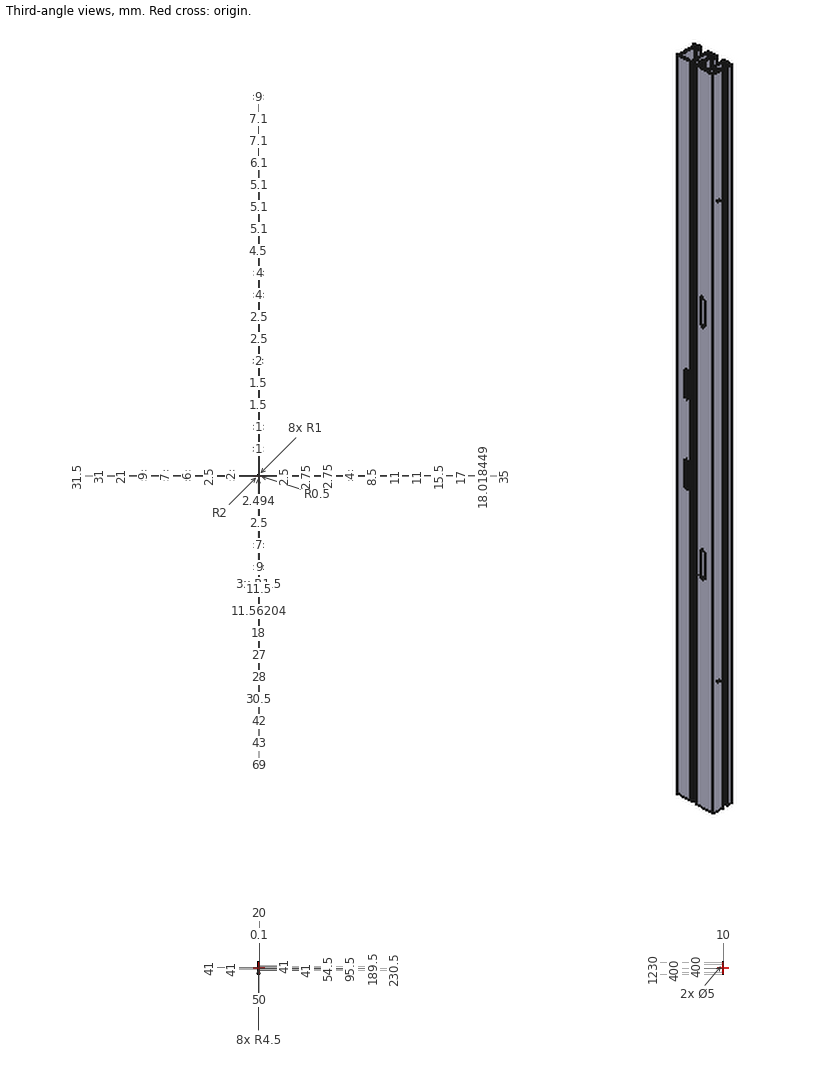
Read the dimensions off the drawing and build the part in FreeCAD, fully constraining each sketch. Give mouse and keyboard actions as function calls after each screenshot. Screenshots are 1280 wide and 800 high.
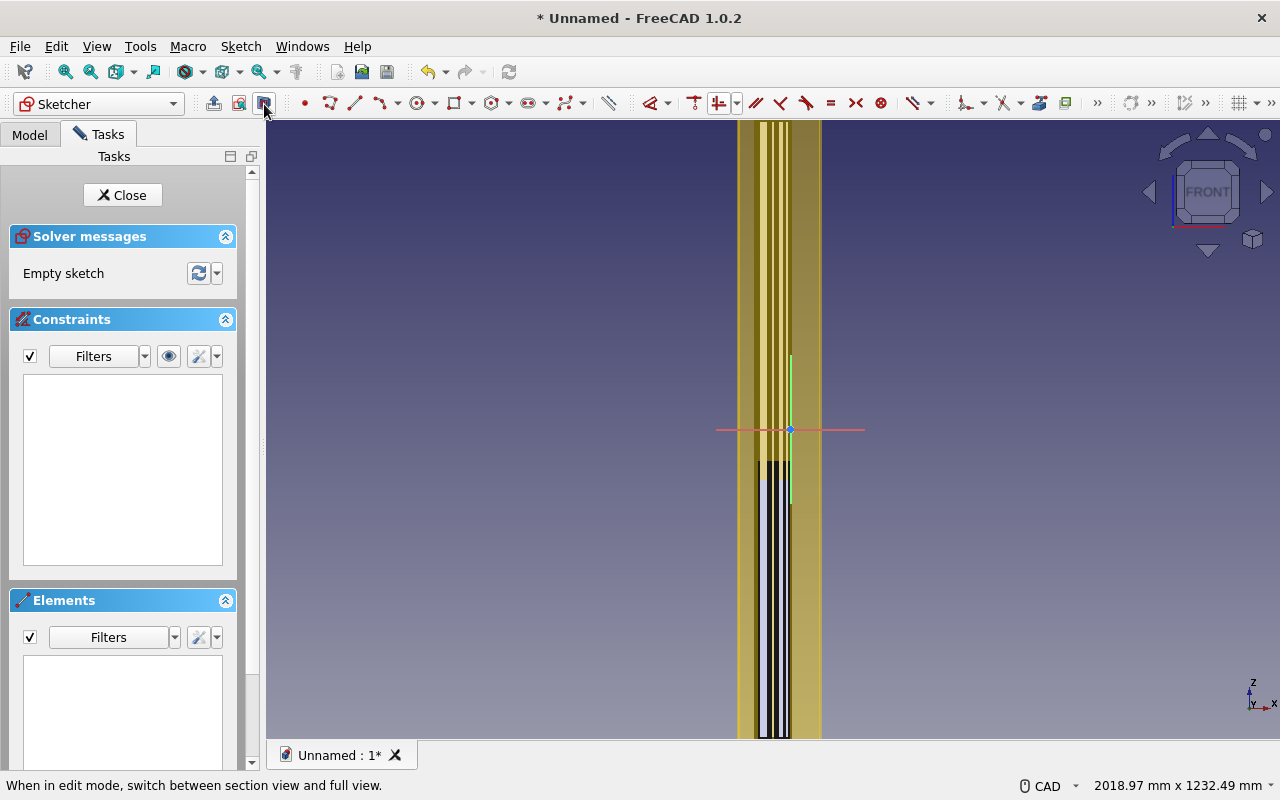
scroll(865, 430, up, 3)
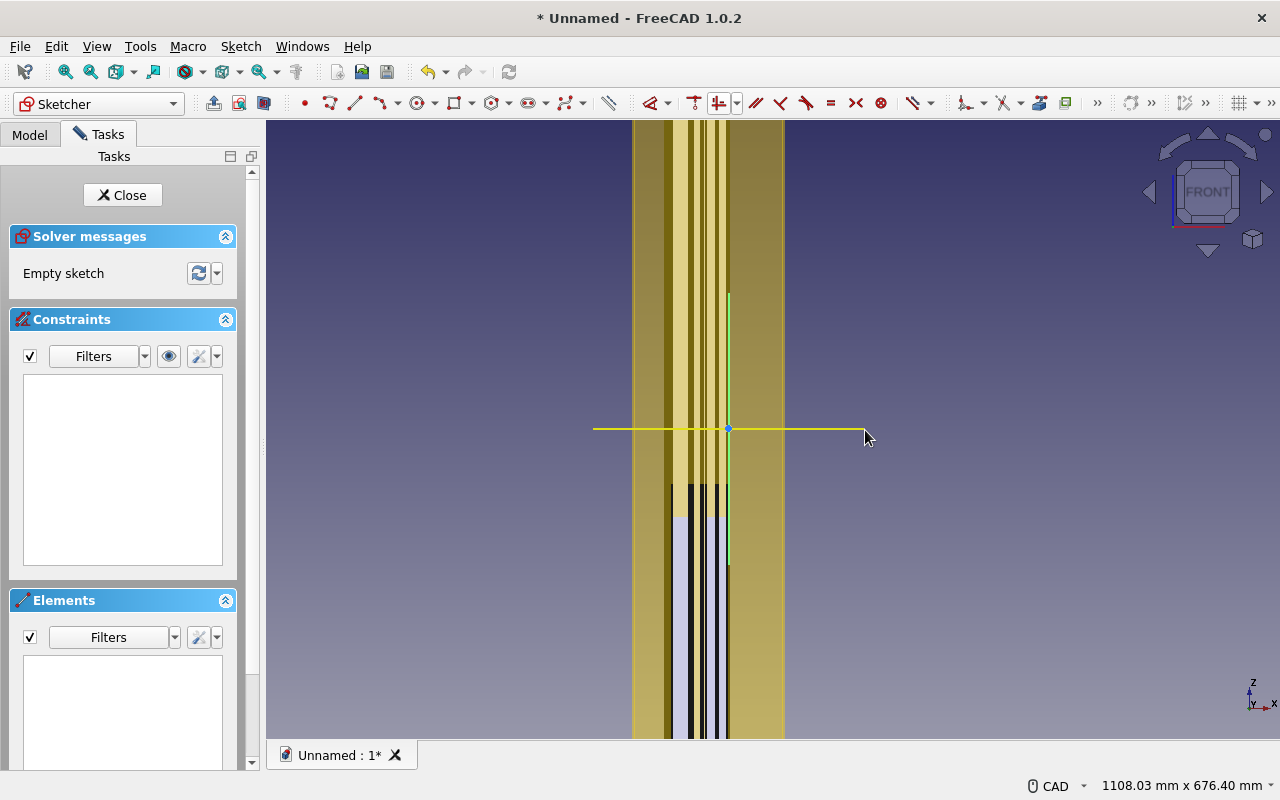
click(528, 104)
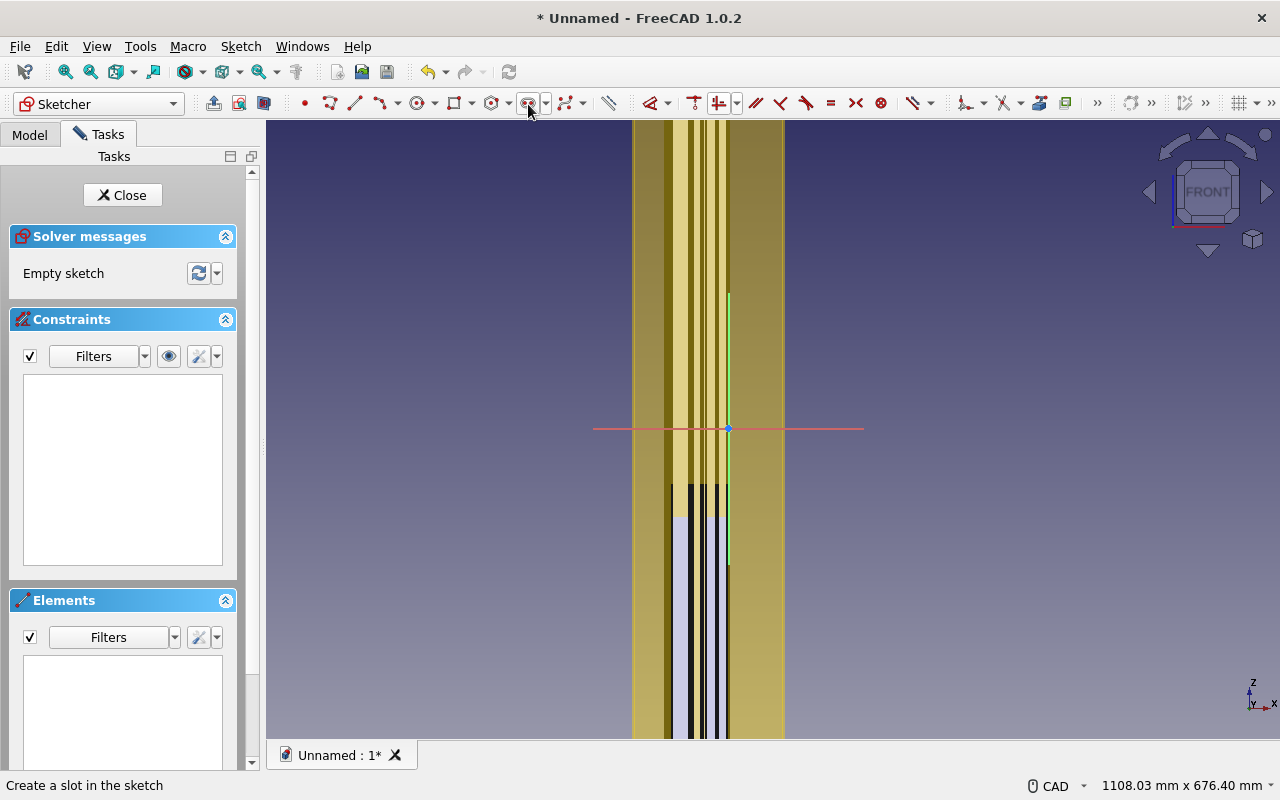
scroll(711, 255, up, 9)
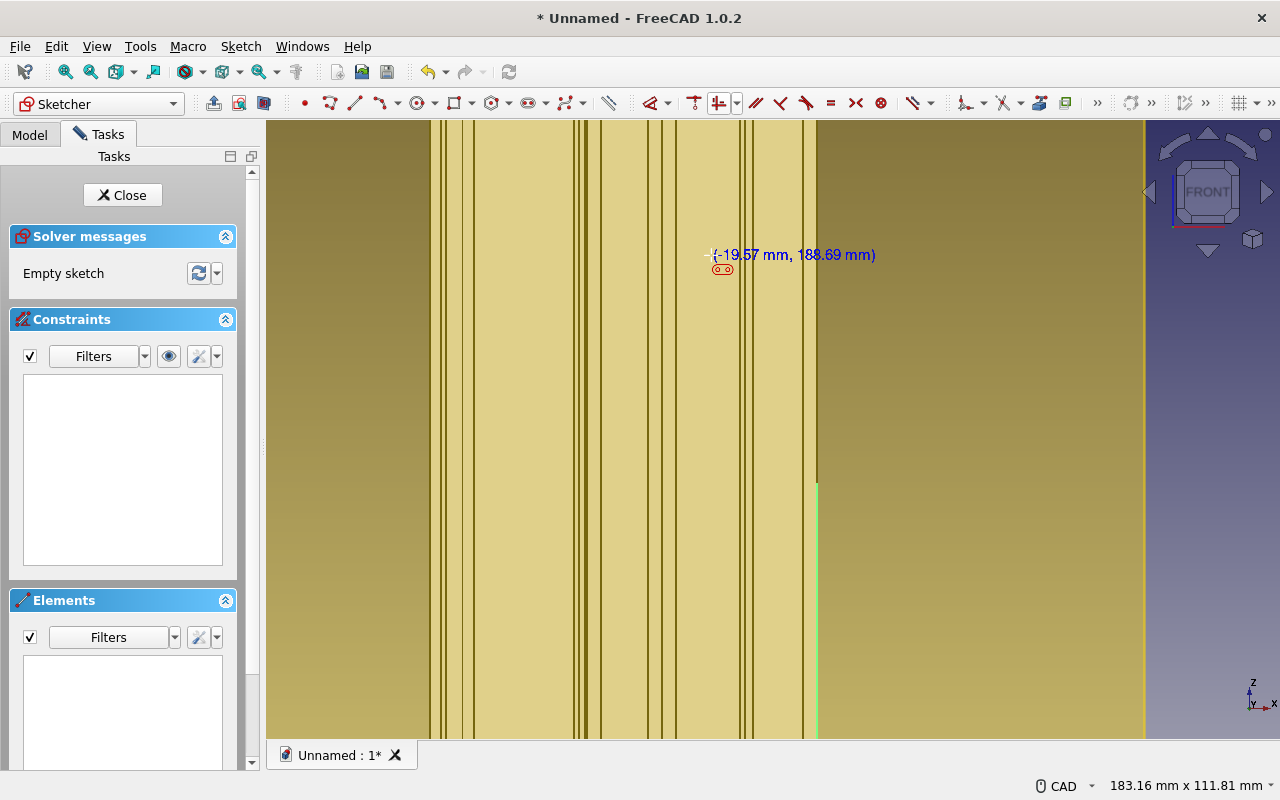
scroll(712, 256, down, 9)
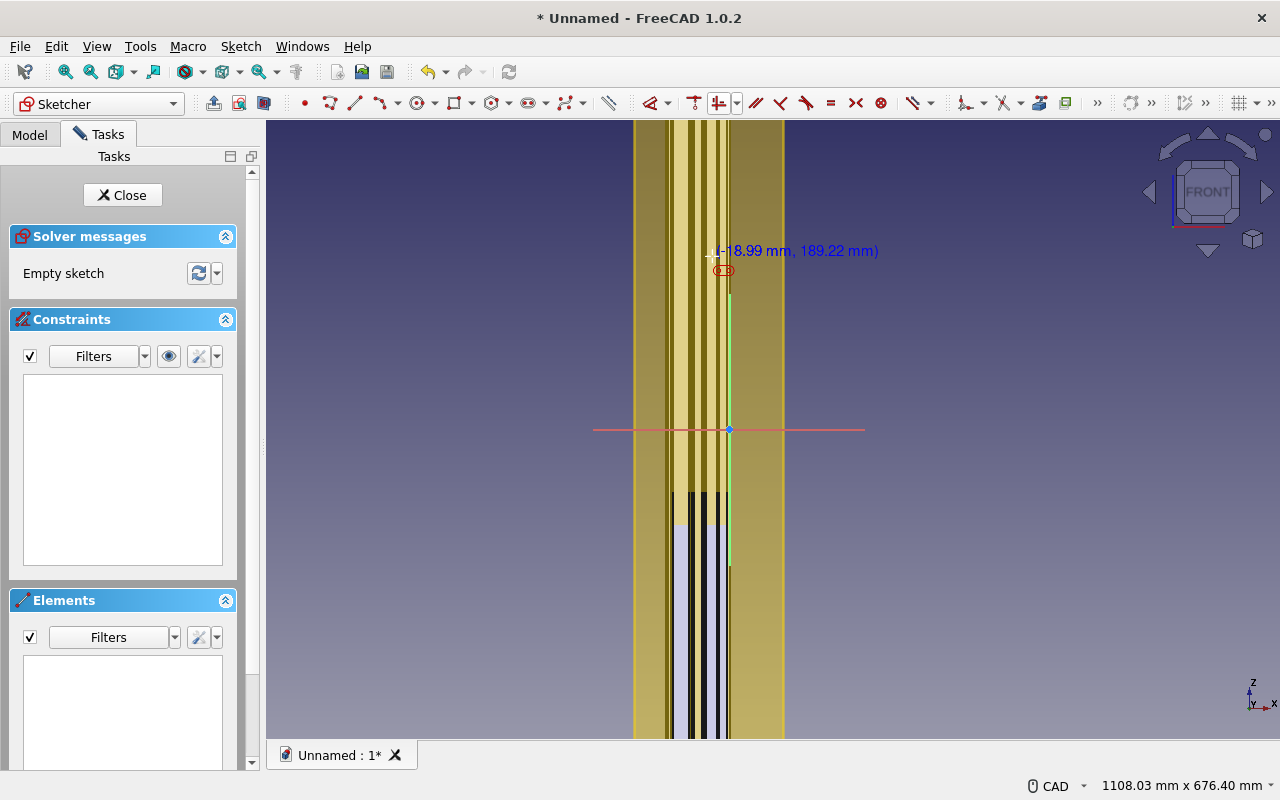
click(711, 256)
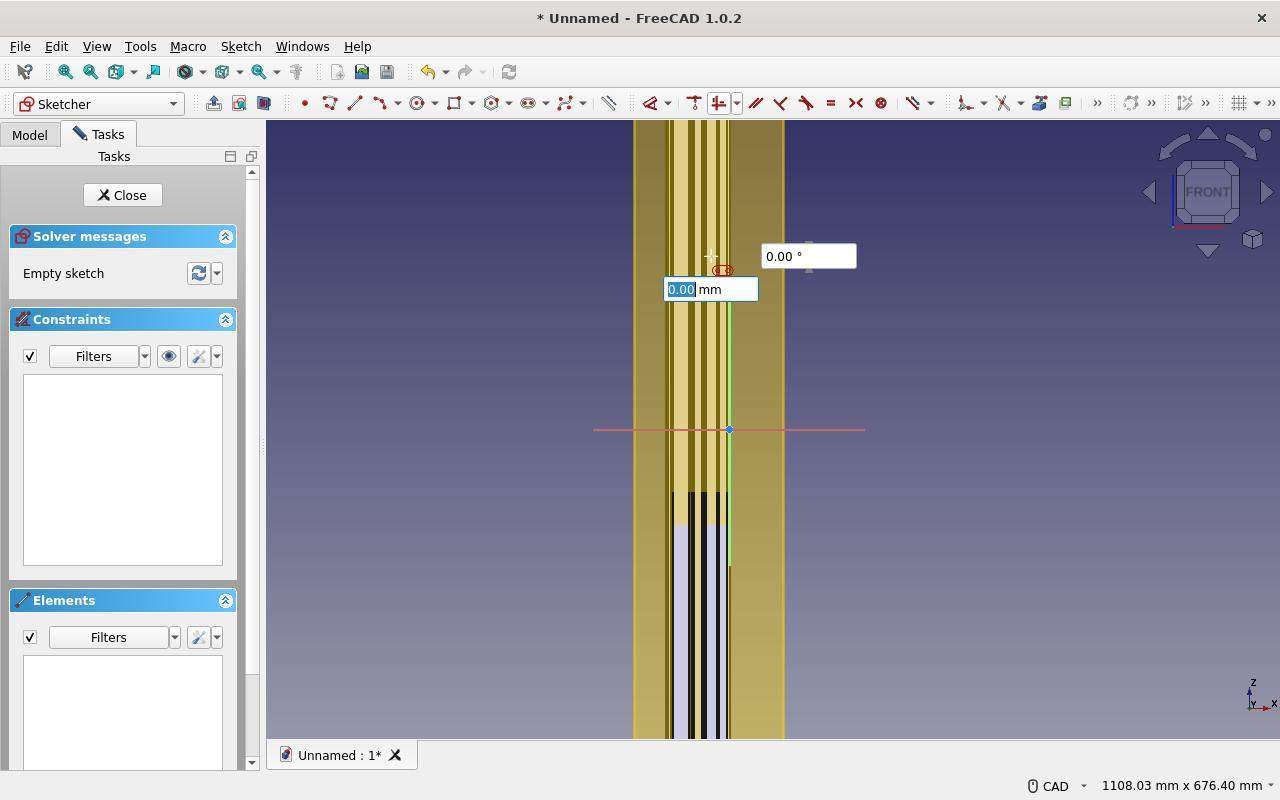
click(711, 219)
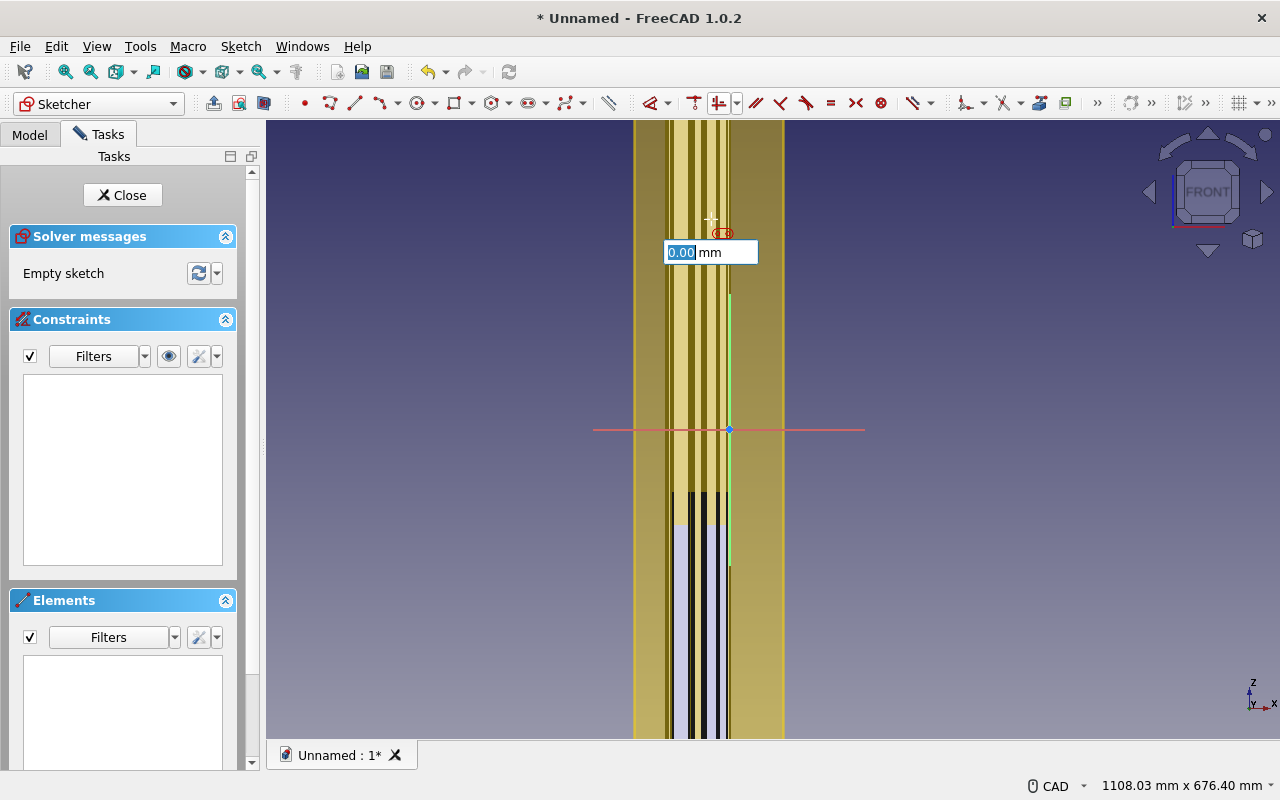
scroll(716, 237, up, 7)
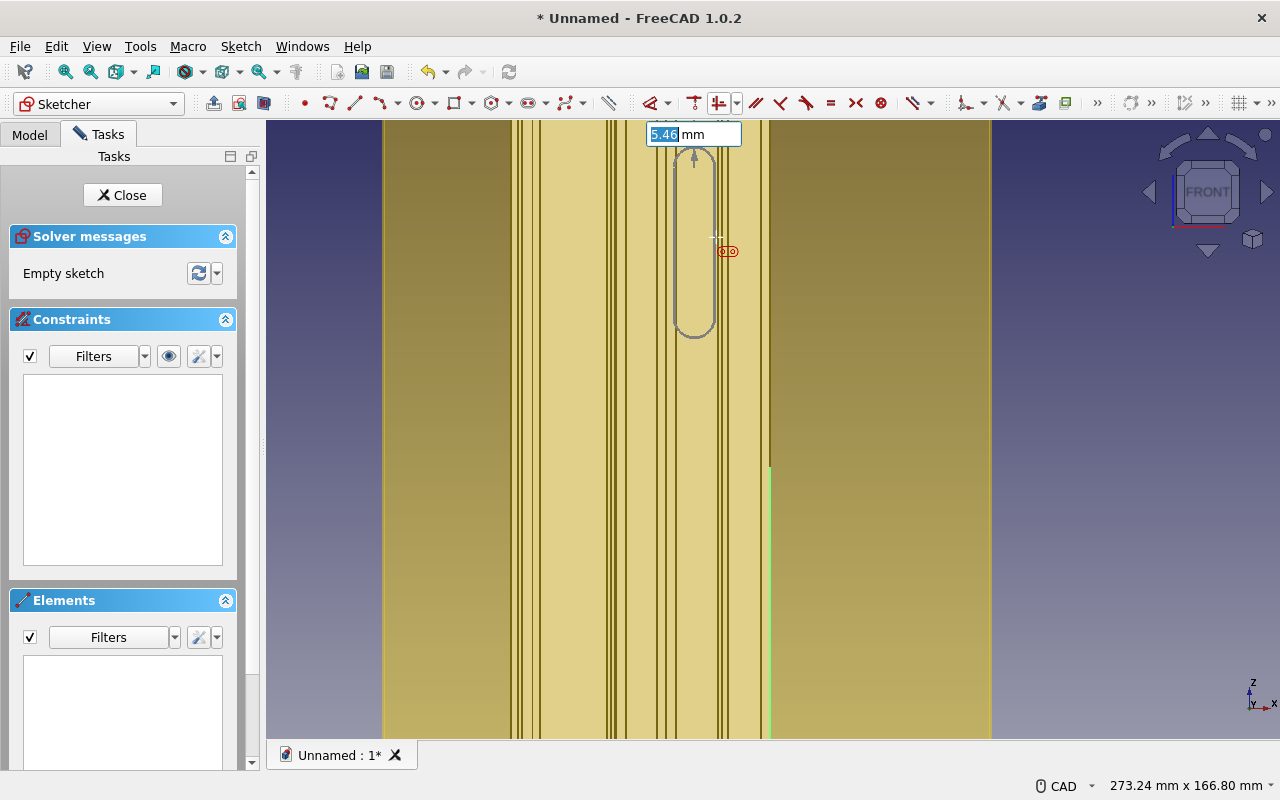
click(713, 238)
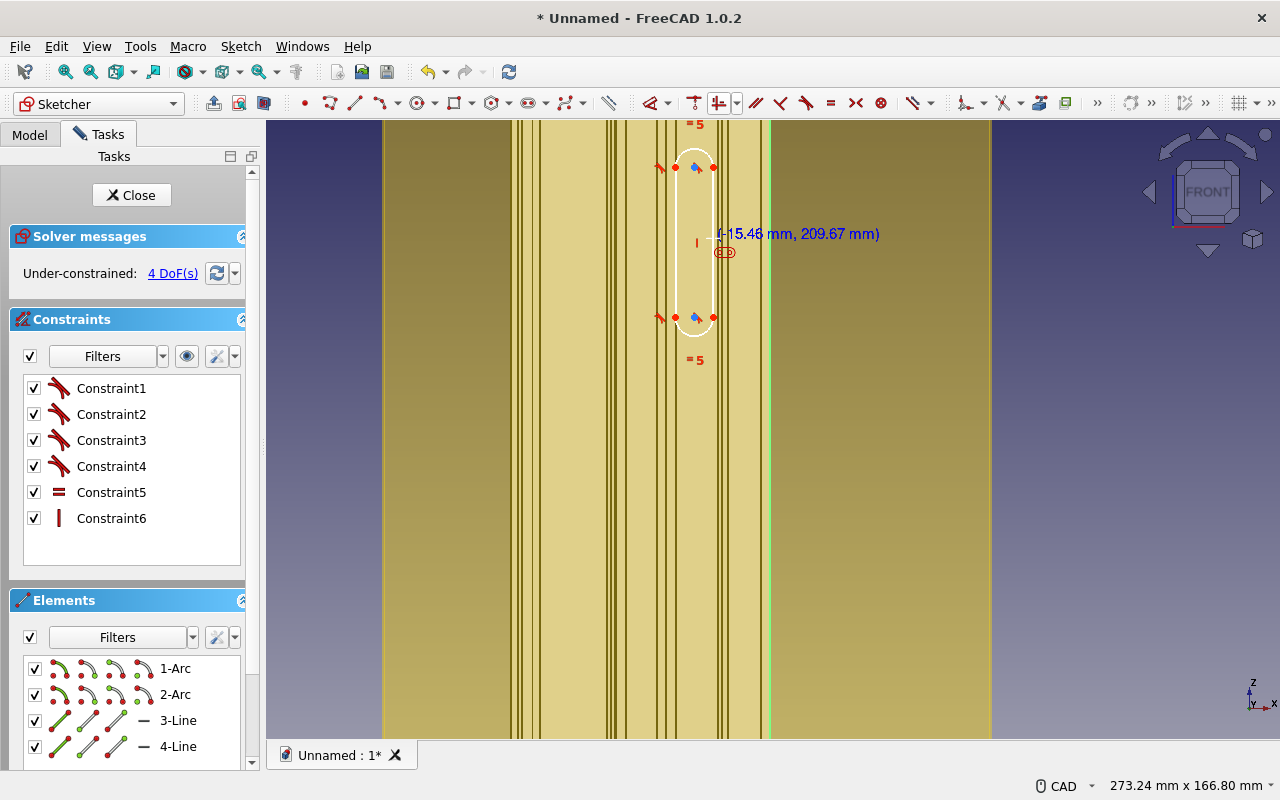
scroll(716, 237, down, 7)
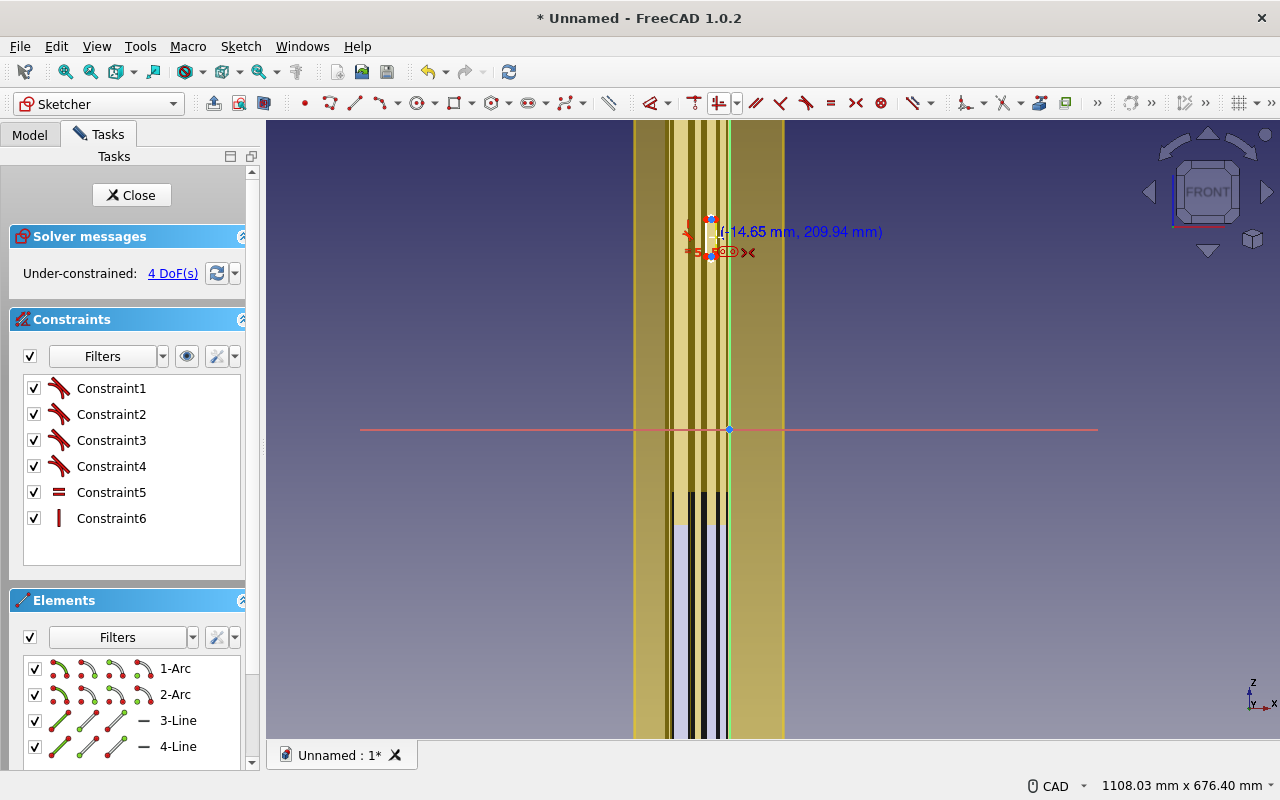
scroll(684, 517, up, 9)